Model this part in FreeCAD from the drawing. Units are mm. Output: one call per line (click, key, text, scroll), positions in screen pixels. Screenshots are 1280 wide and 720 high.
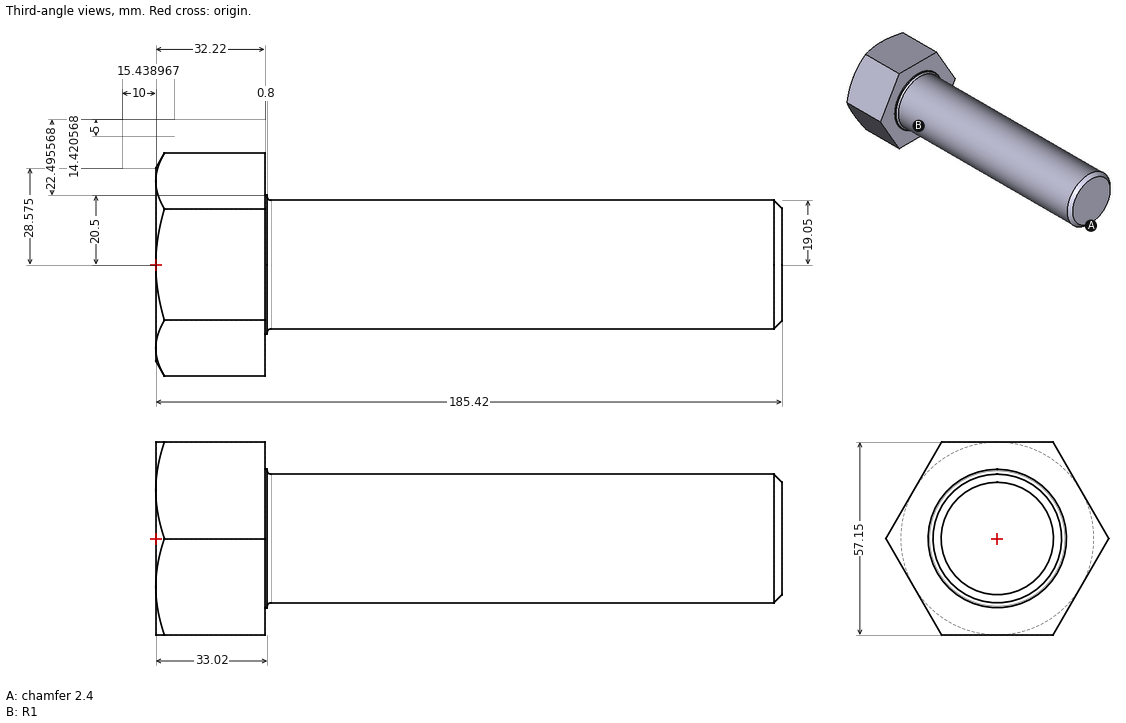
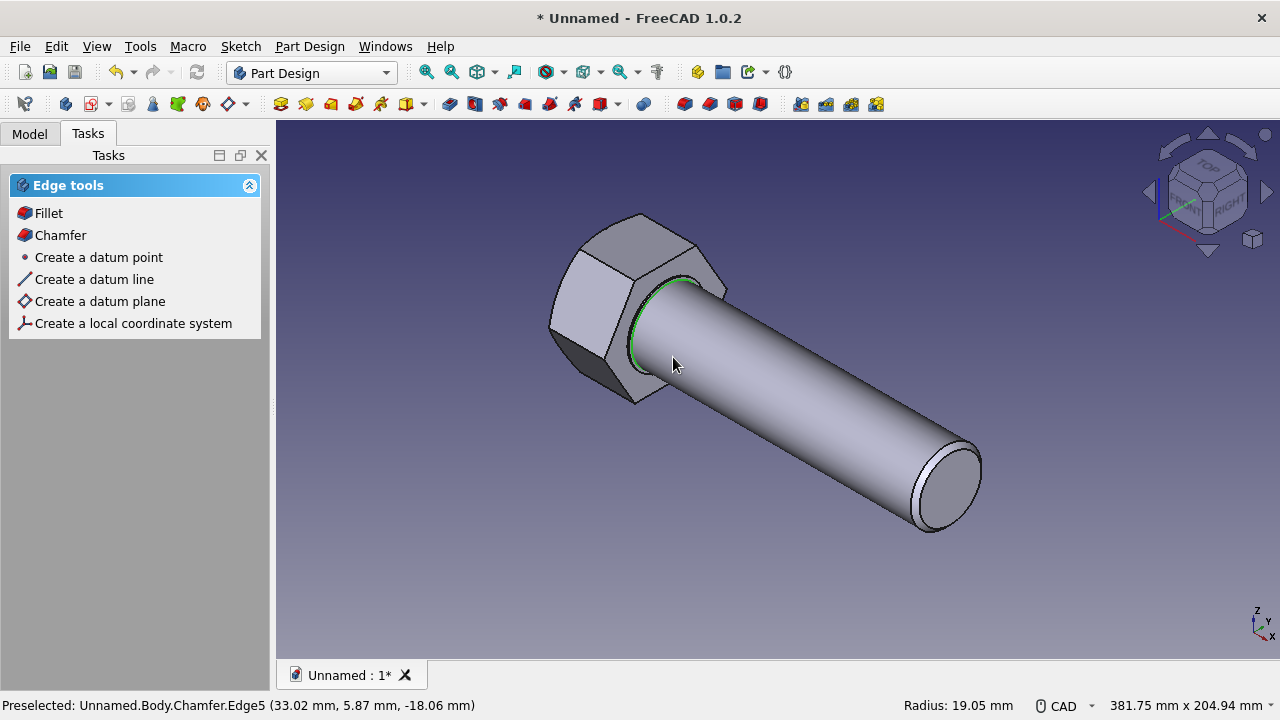
click(685, 104)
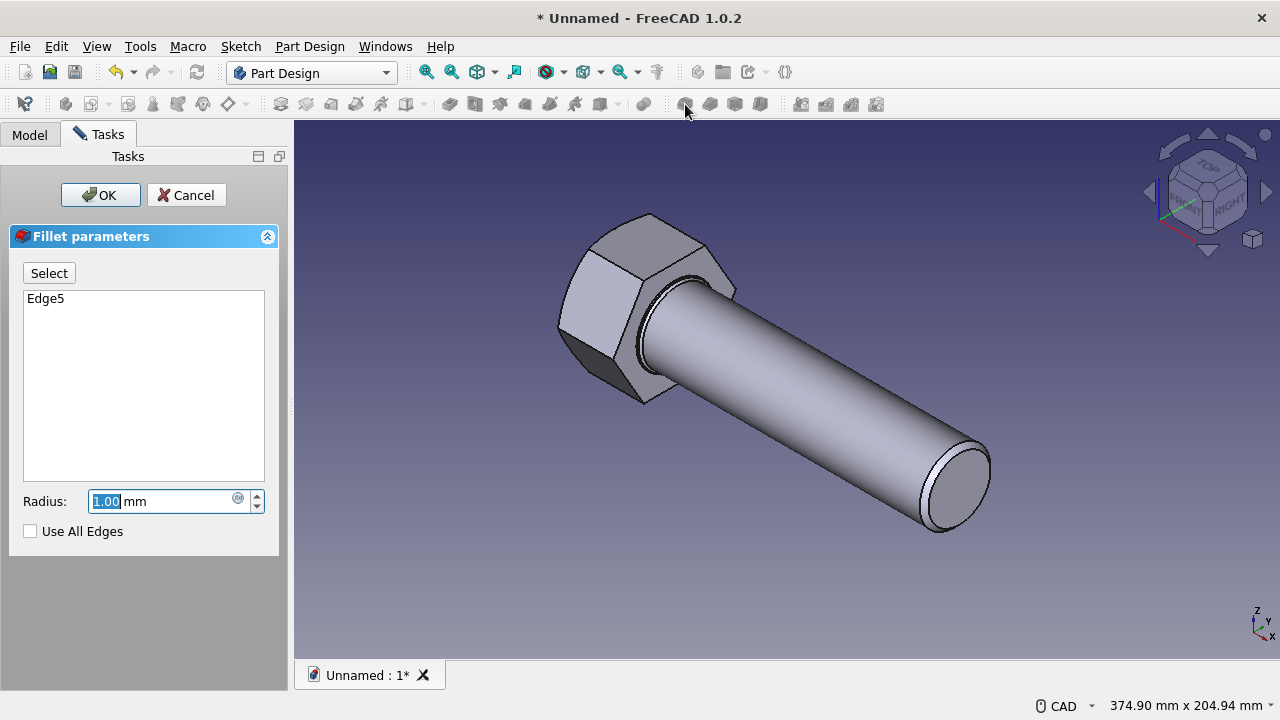
text(1)
key(Tab)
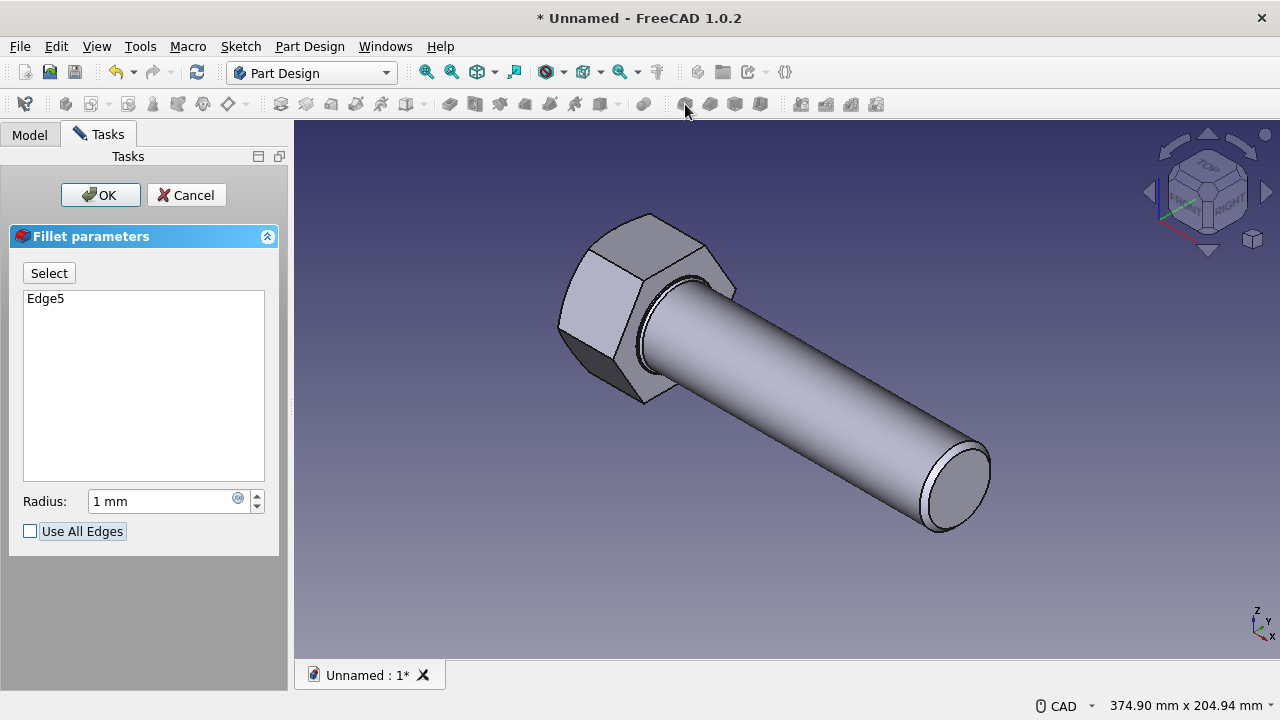
click(101, 195)